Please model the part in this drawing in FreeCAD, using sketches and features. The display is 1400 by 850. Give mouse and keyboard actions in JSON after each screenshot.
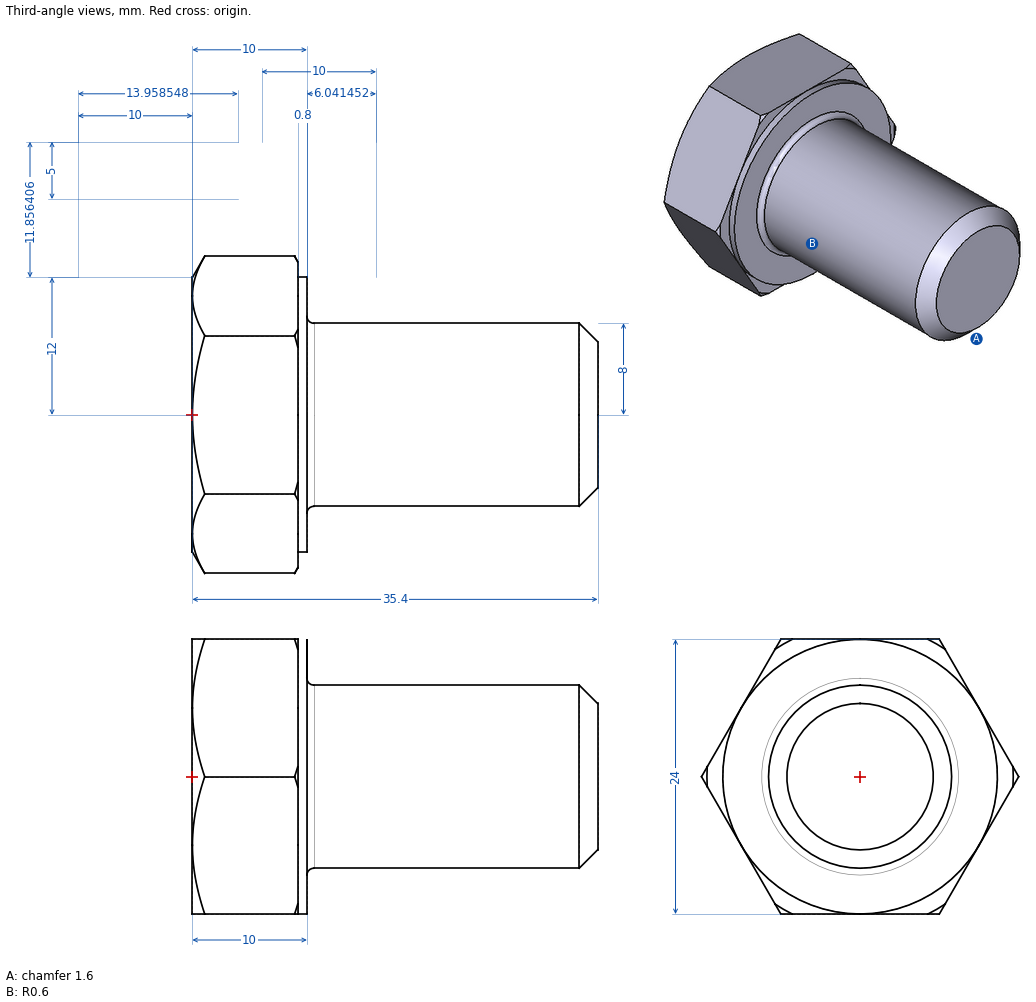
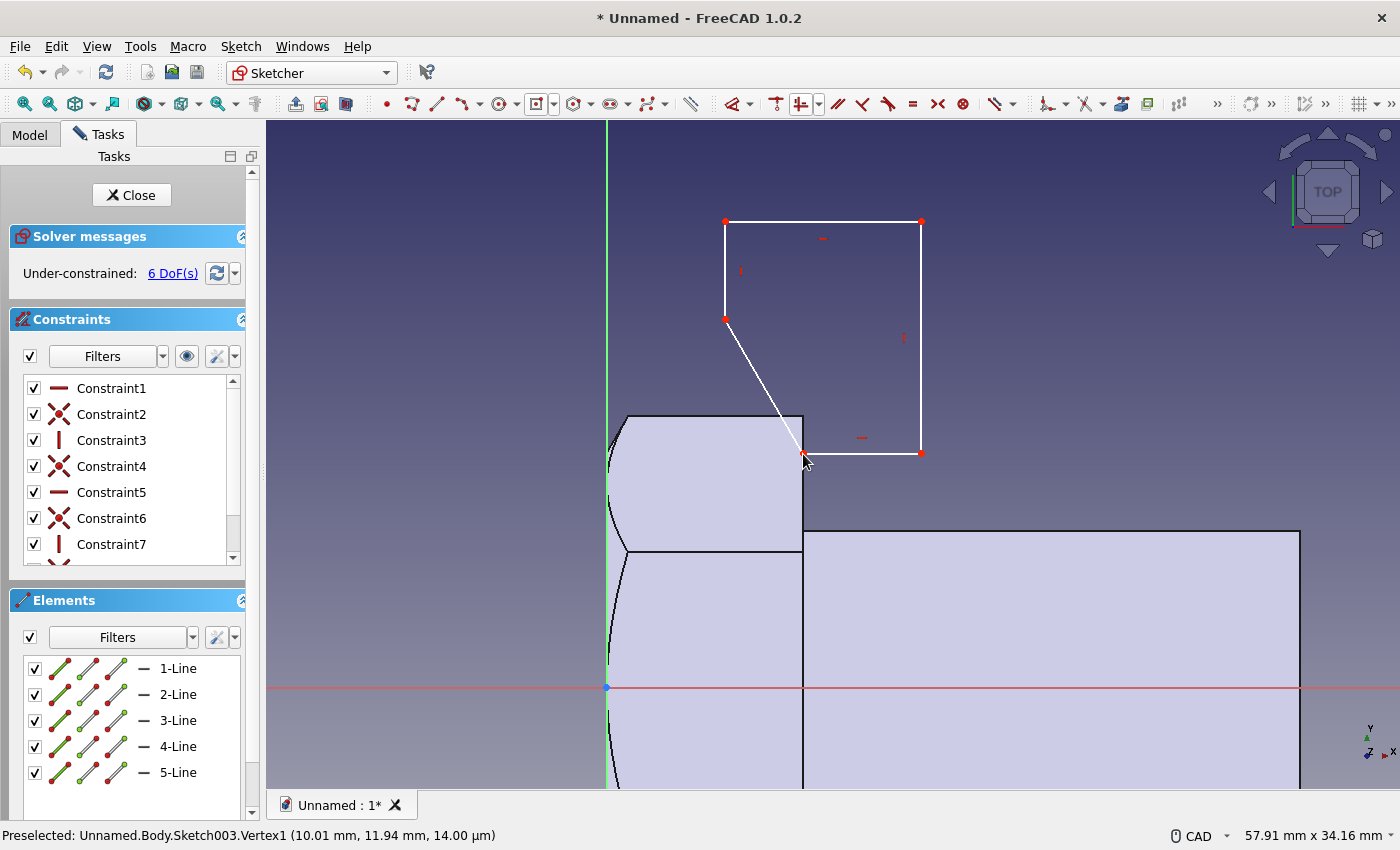
{"action": "key", "text": "d"}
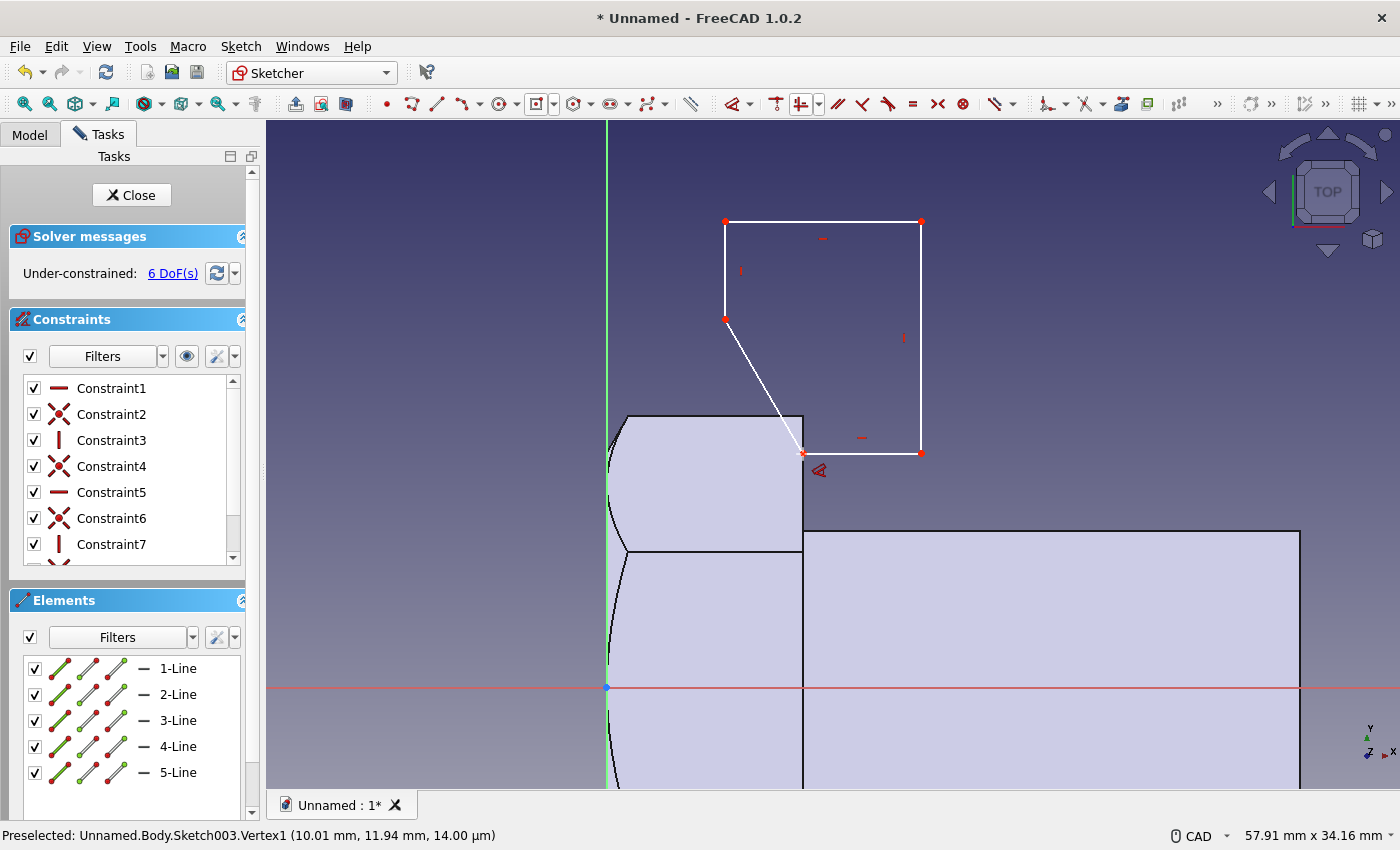
{"action": "left_click", "coordinate": [725, 251]}
{"action": "left_click", "coordinate": [691, 271]}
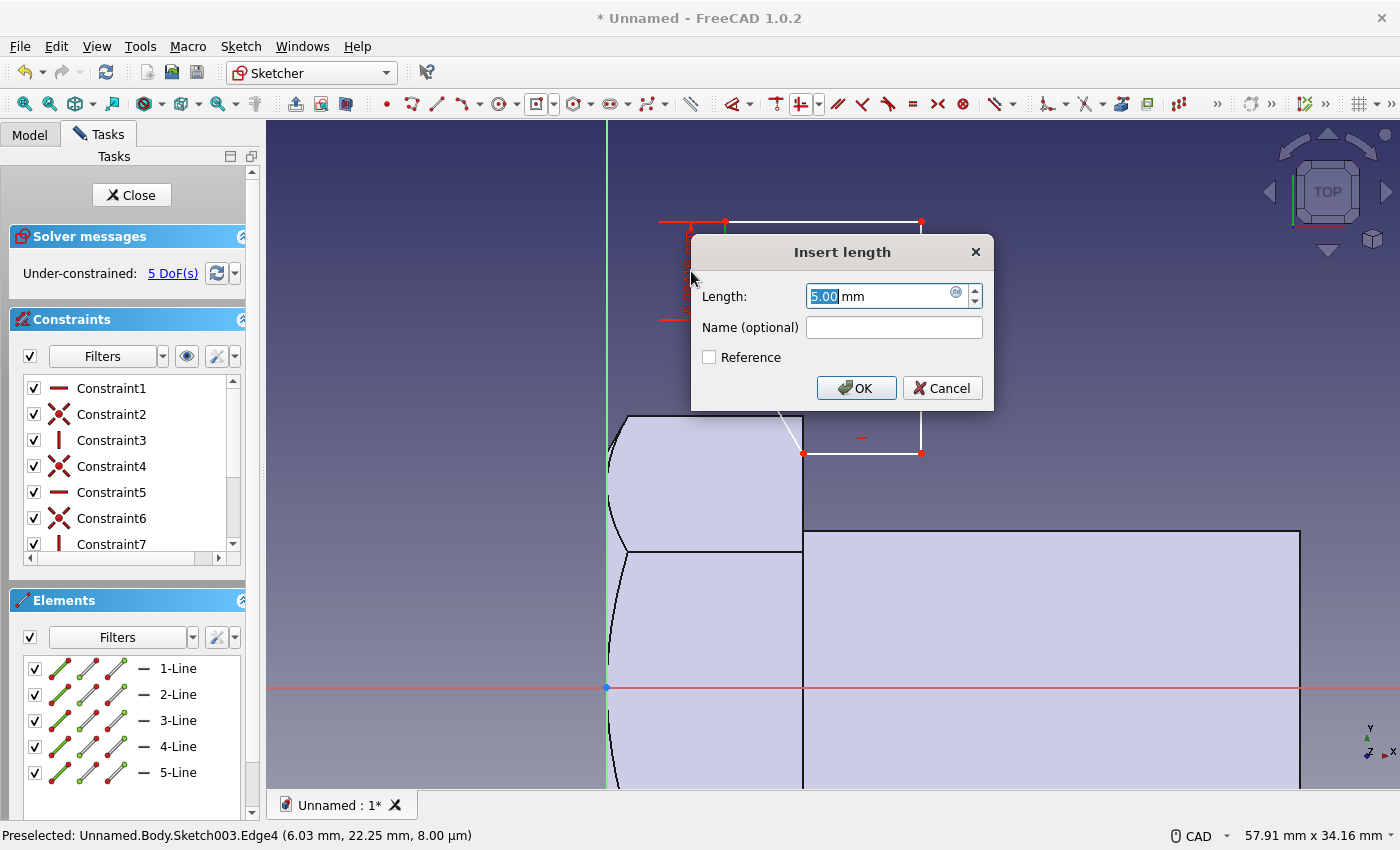
{"action": "type", "text": "5"}
{"action": "key", "text": "Return"}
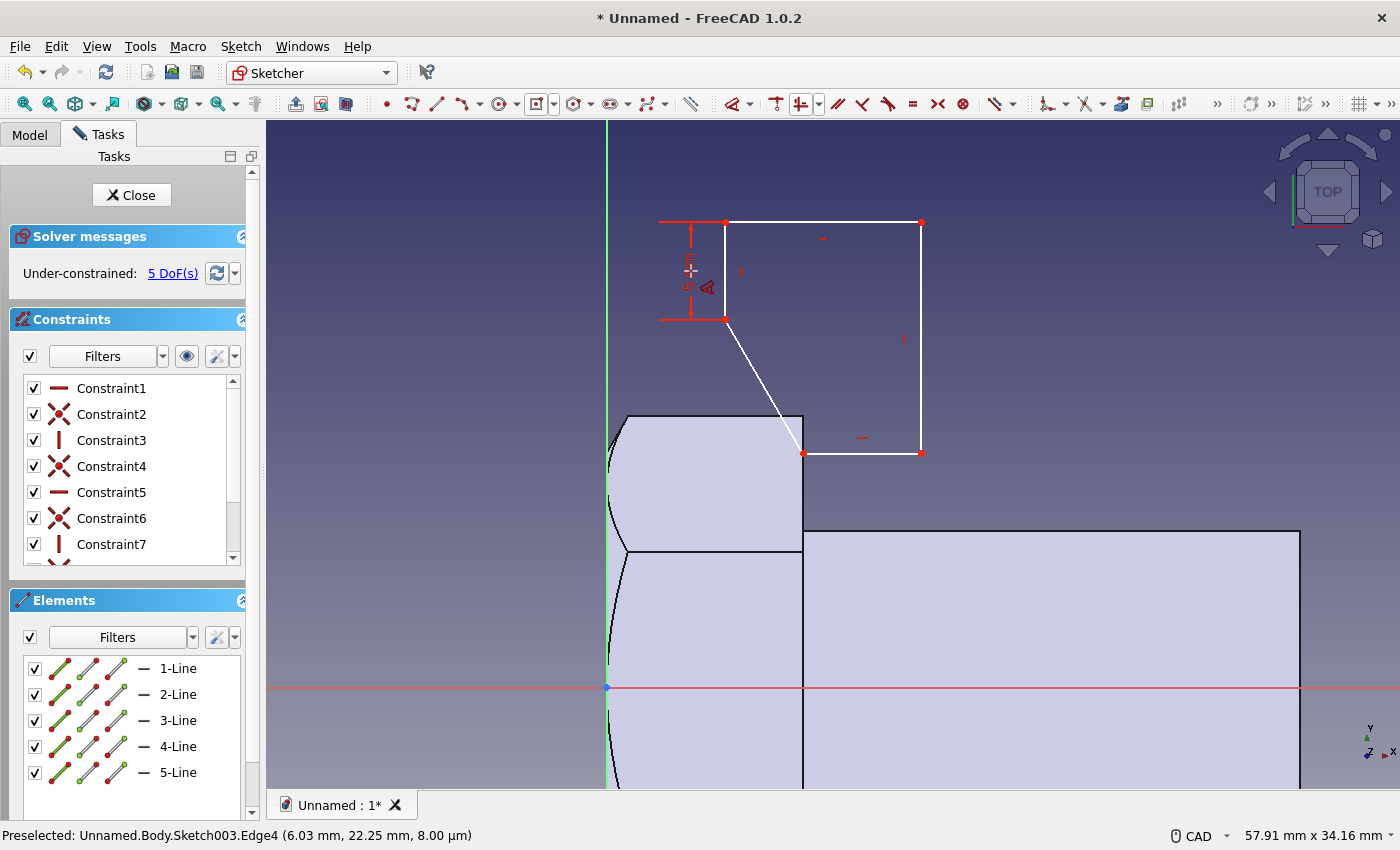
{"action": "left_click", "coordinate": [862, 222]}
{"action": "left_click", "coordinate": [823, 188]}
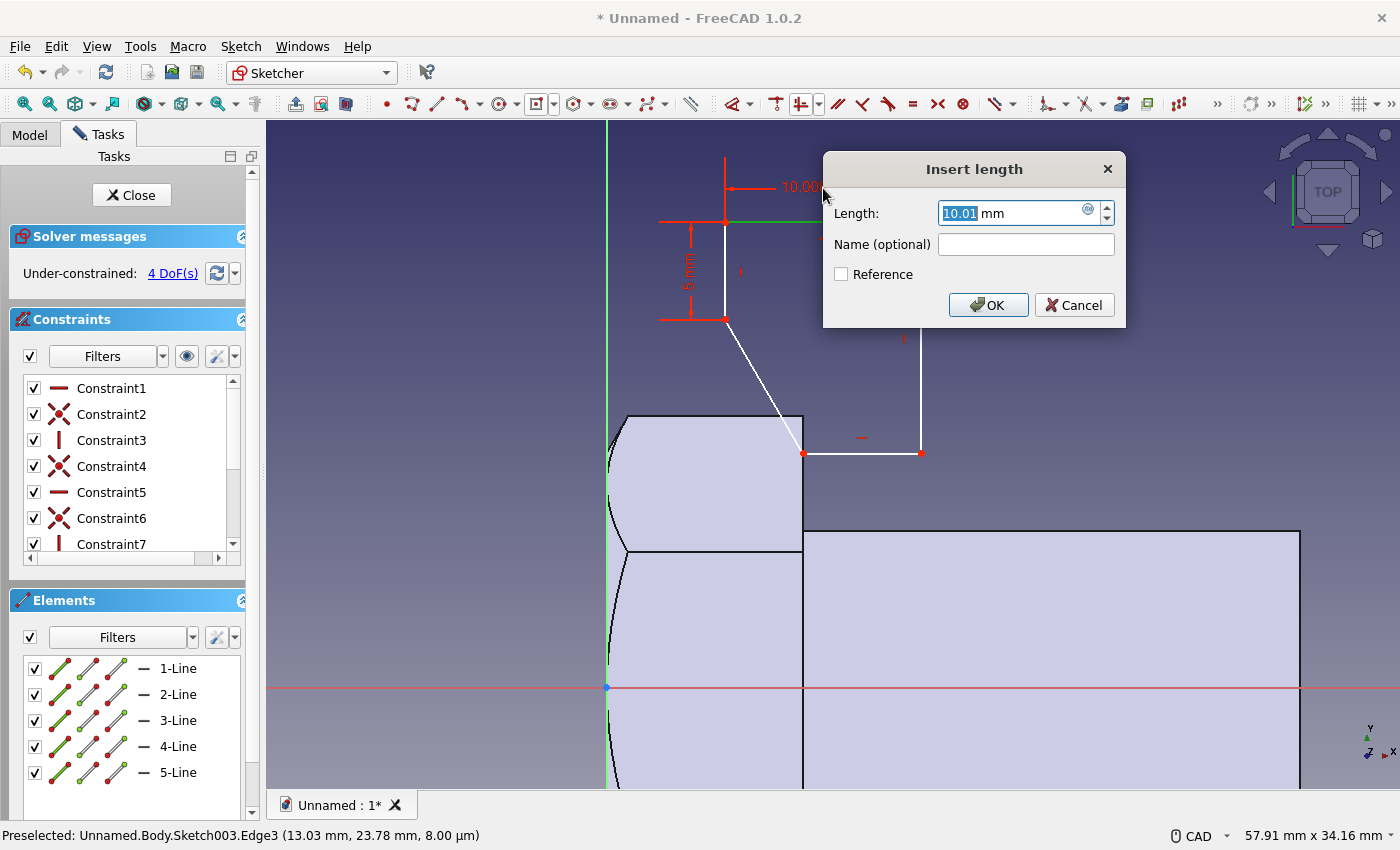
{"action": "type", "text": "10"}
{"action": "key", "text": "Return"}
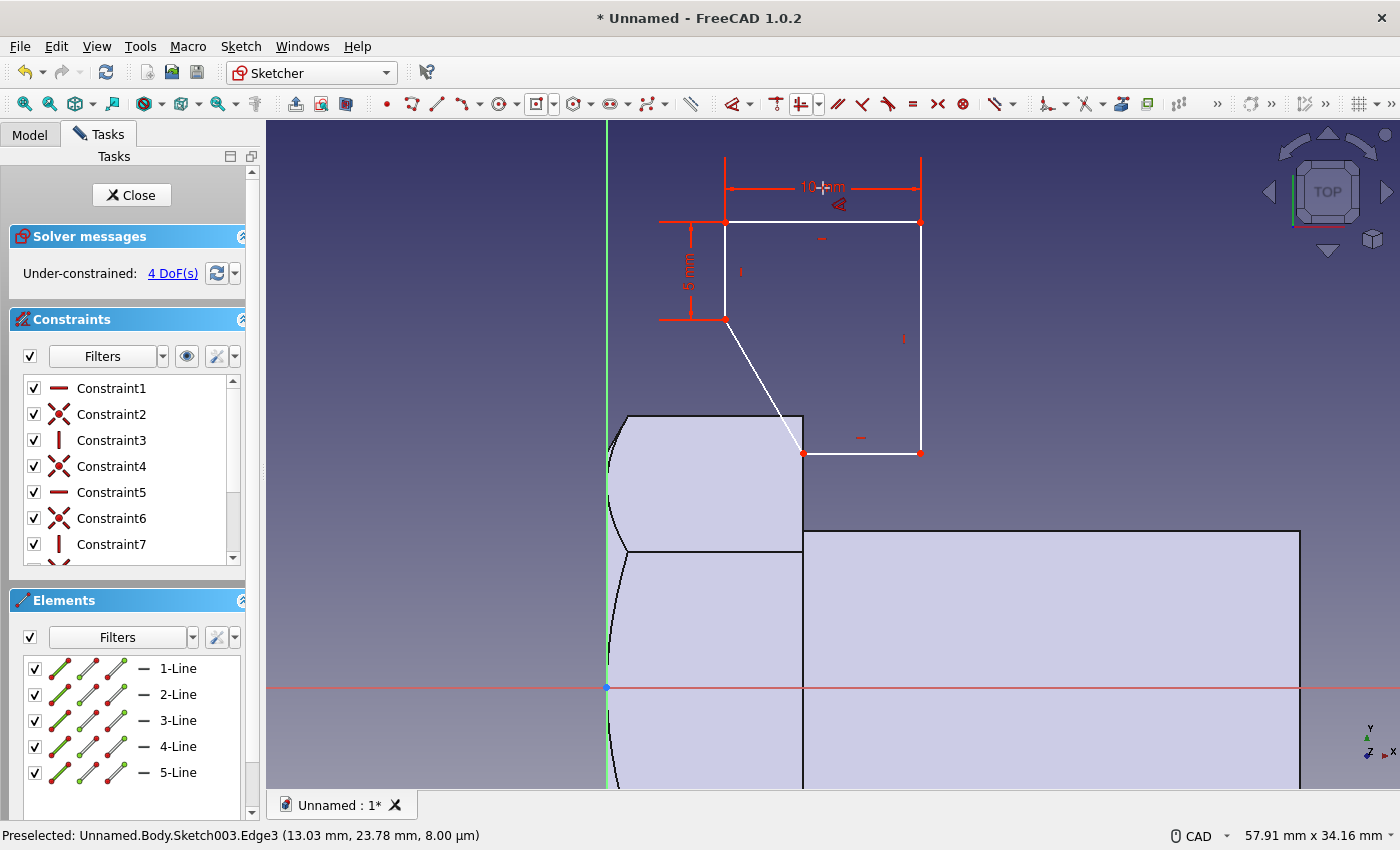
{"action": "left_click", "coordinate": [803, 454]}
{"action": "left_click", "coordinate": [705, 722]}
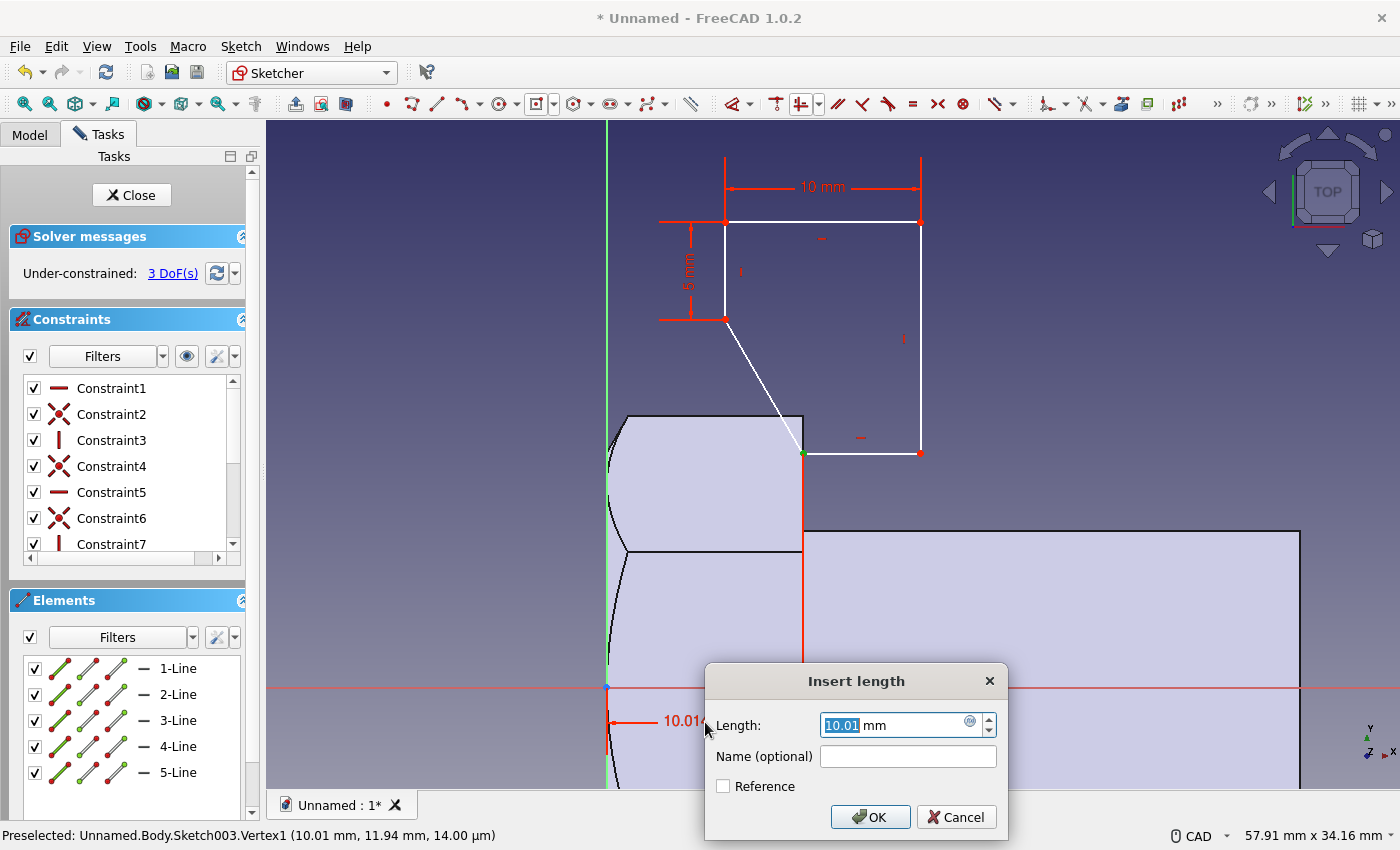
{"action": "type", "text": "10"}
{"action": "key", "text": "Return"}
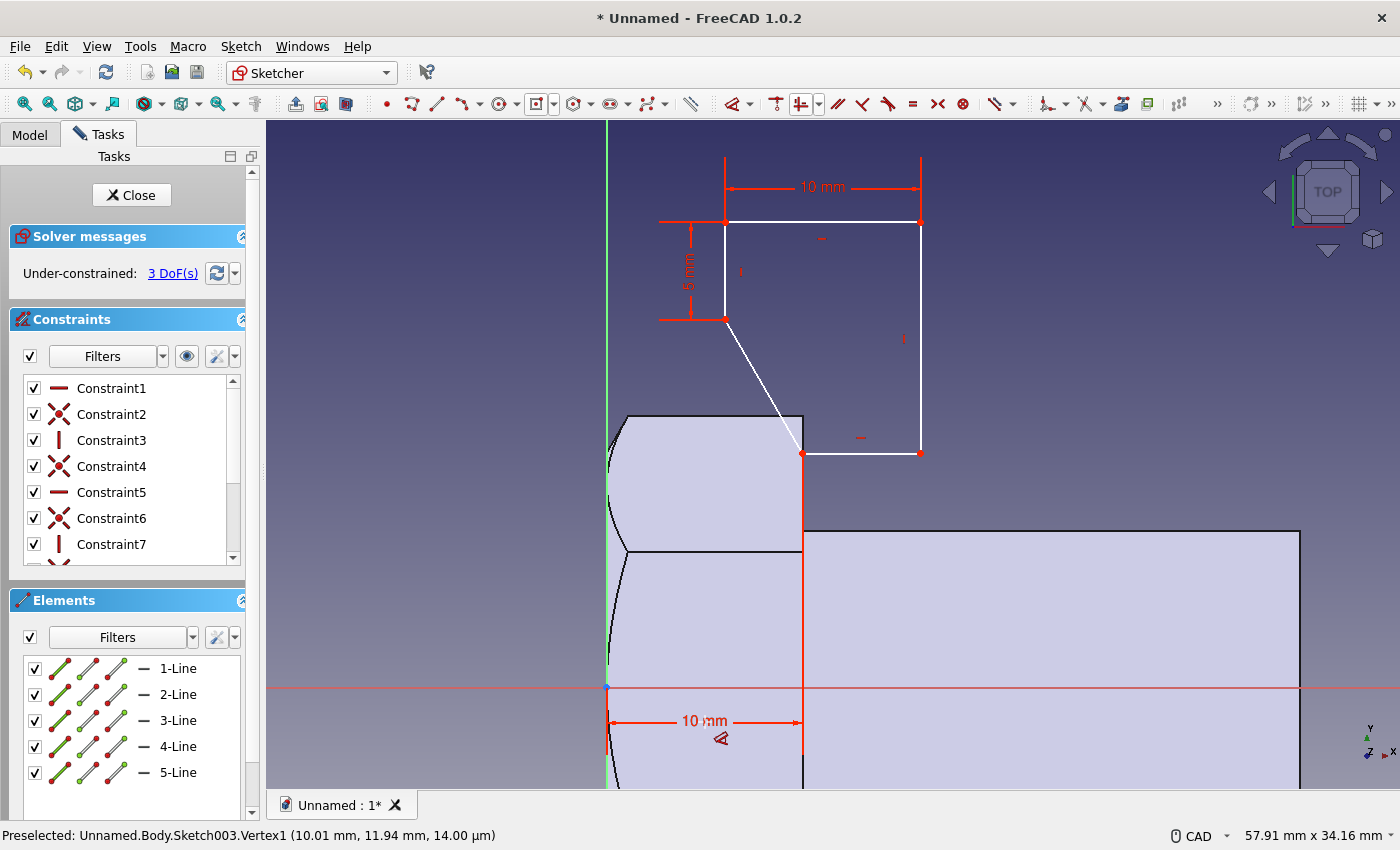
{"action": "left_click", "coordinate": [803, 454]}
{"action": "left_click", "coordinate": [573, 571]}